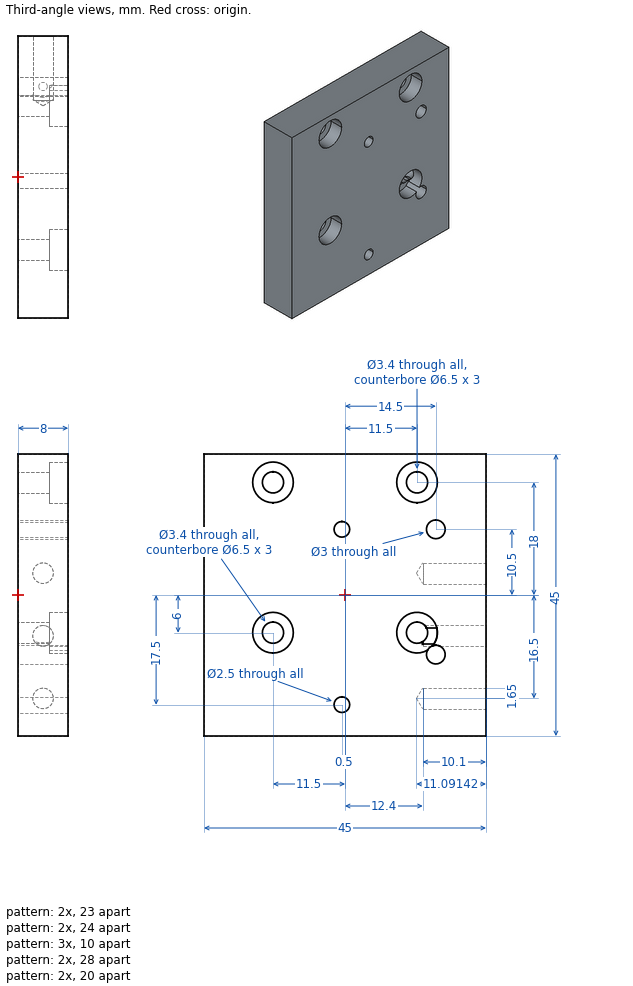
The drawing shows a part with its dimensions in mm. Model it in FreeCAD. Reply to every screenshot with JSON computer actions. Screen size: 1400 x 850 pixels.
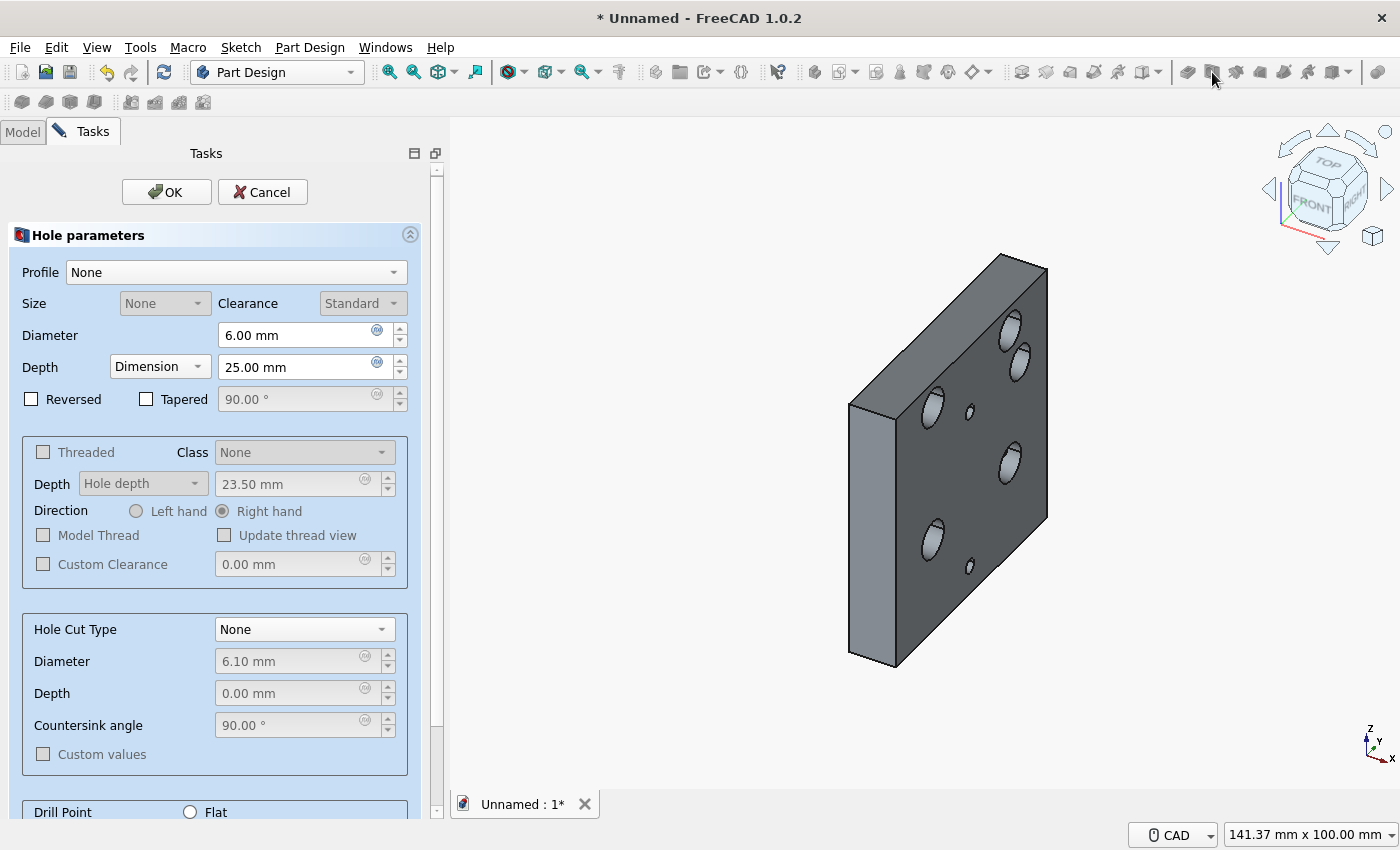
{"action": "triple_click", "coordinate": [305, 335]}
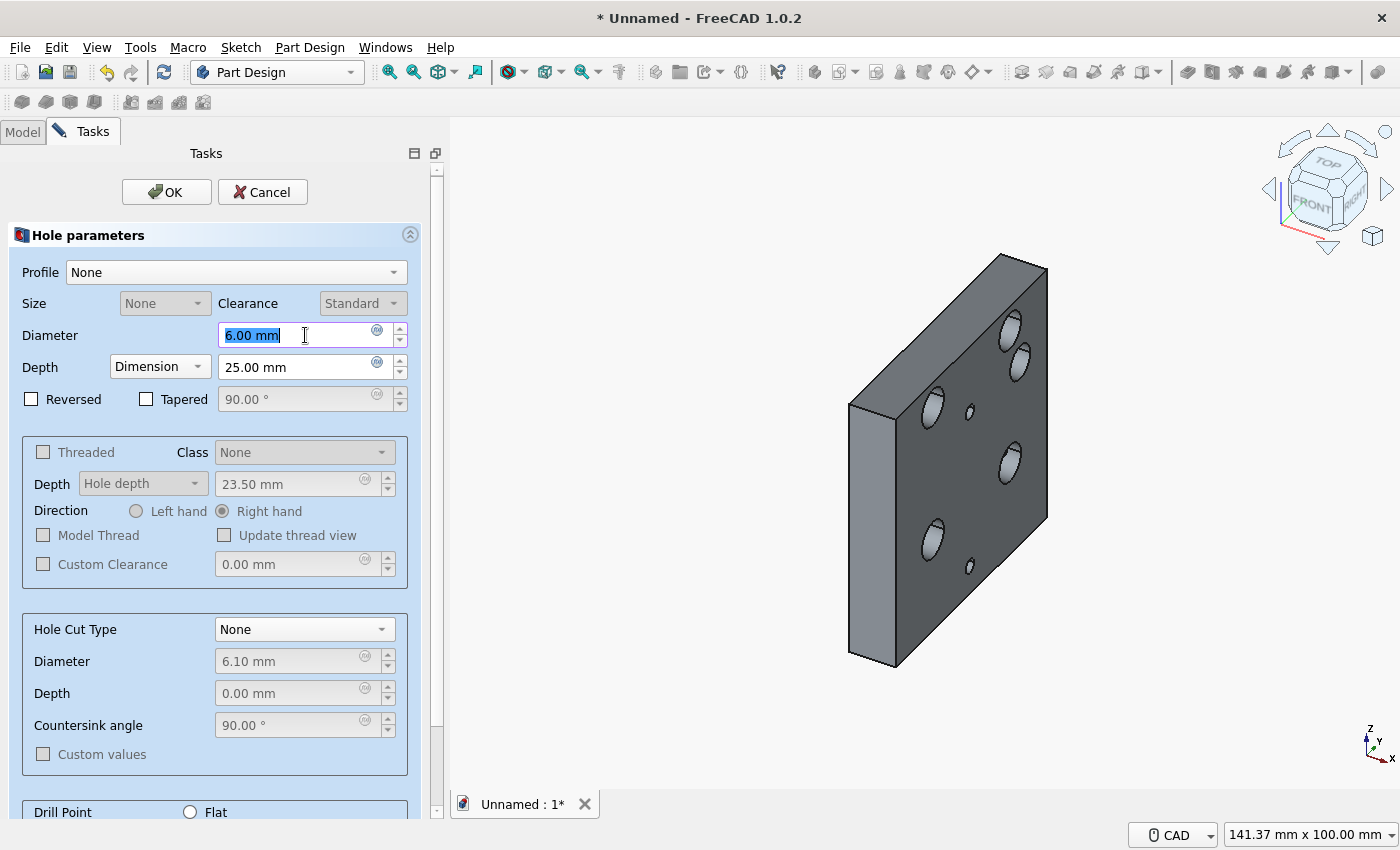
{"action": "type", "text": "3"}
{"action": "key", "text": "Tab"}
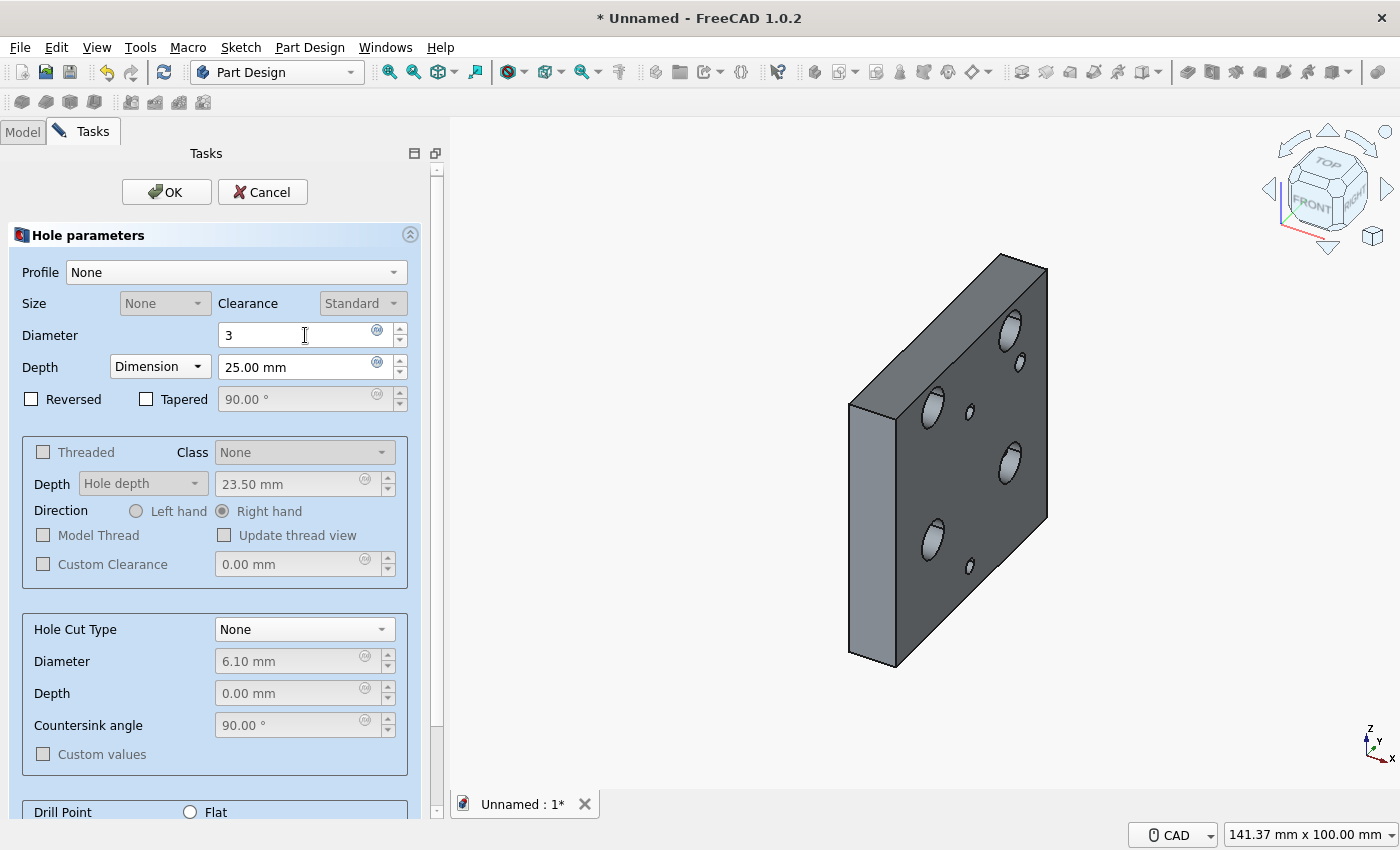
{"action": "left_click", "coordinate": [161, 366]}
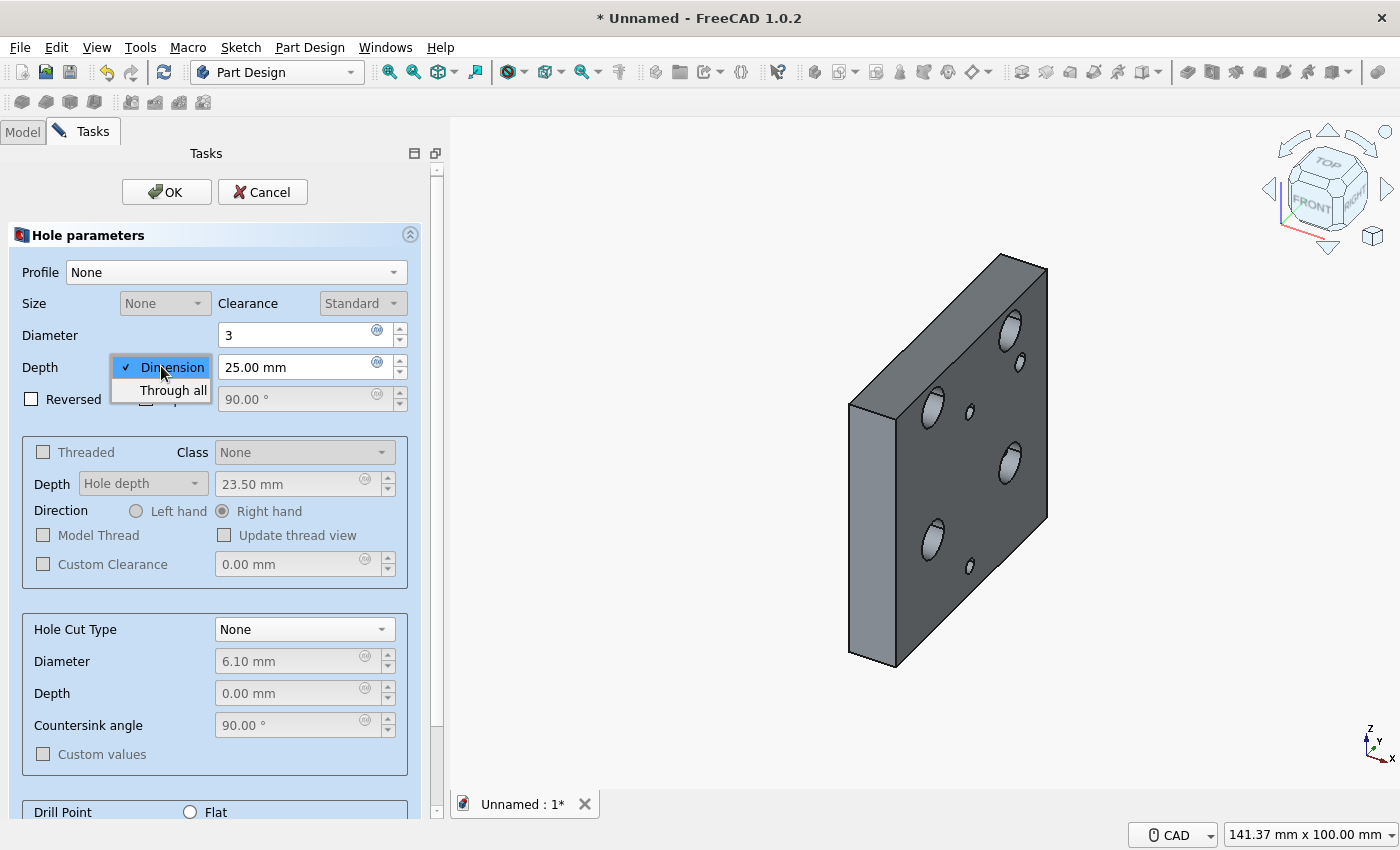
{"action": "left_click", "coordinate": [160, 390]}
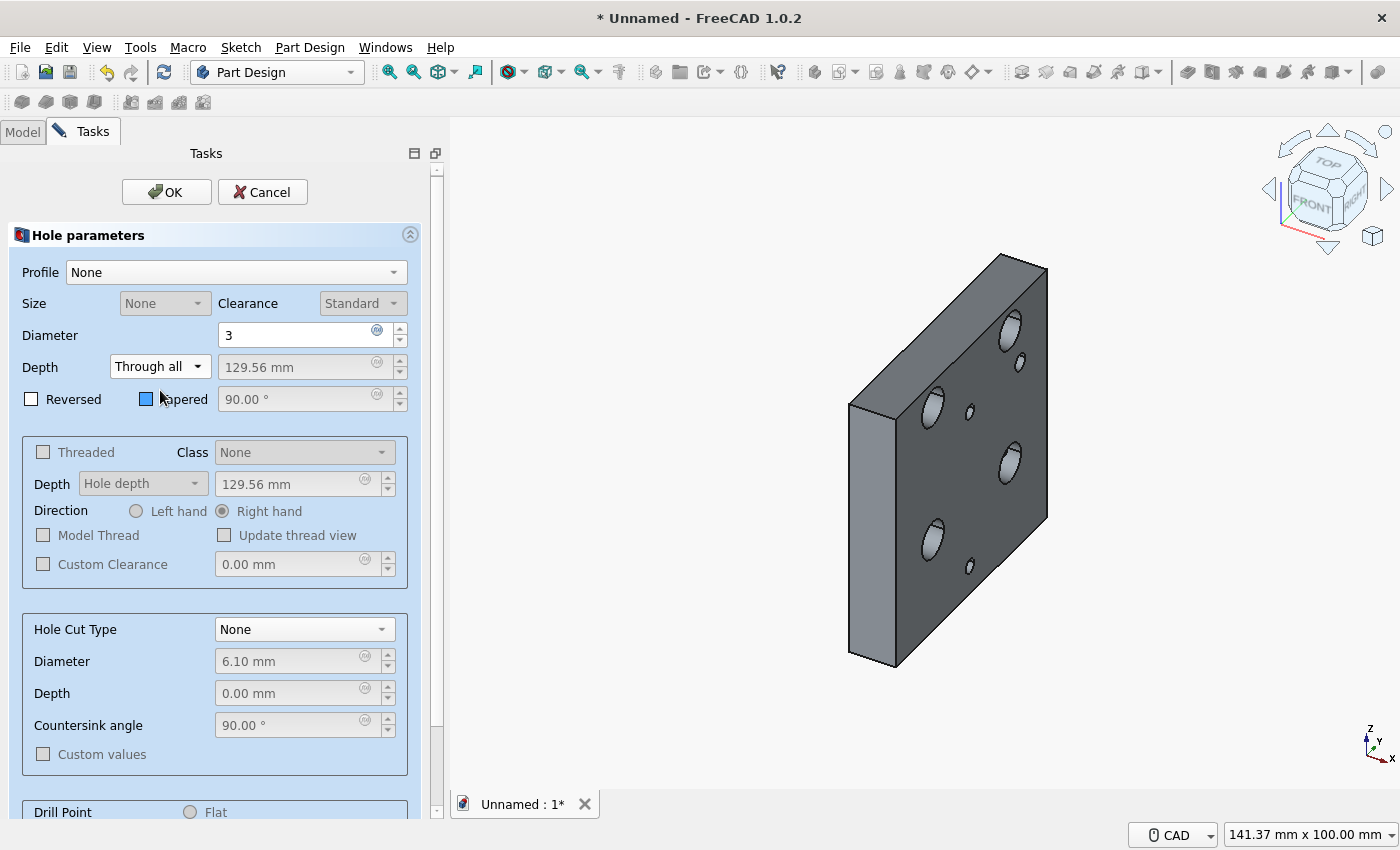
{"action": "left_click", "coordinate": [167, 192]}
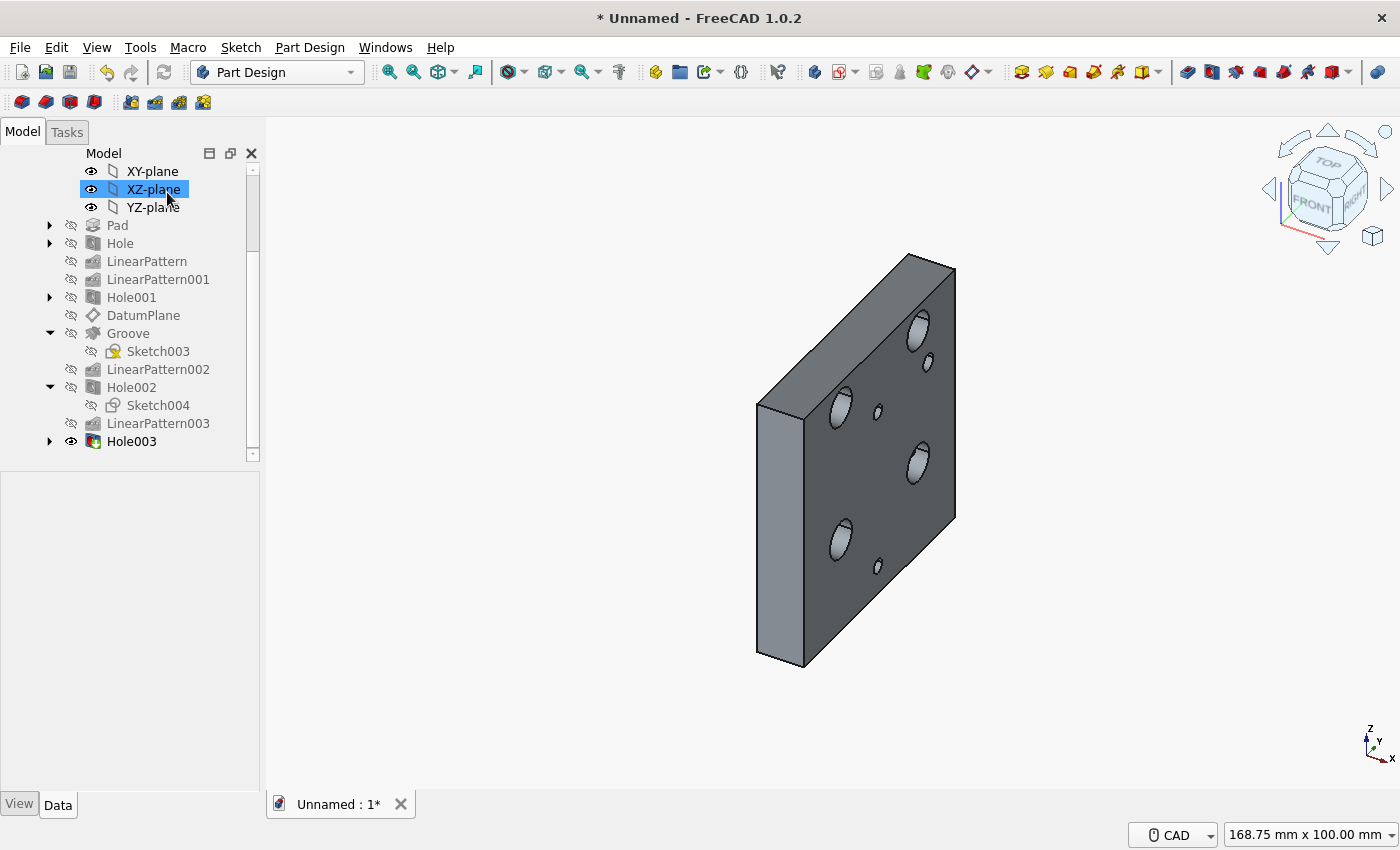
{"action": "left_click", "coordinate": [116, 441]}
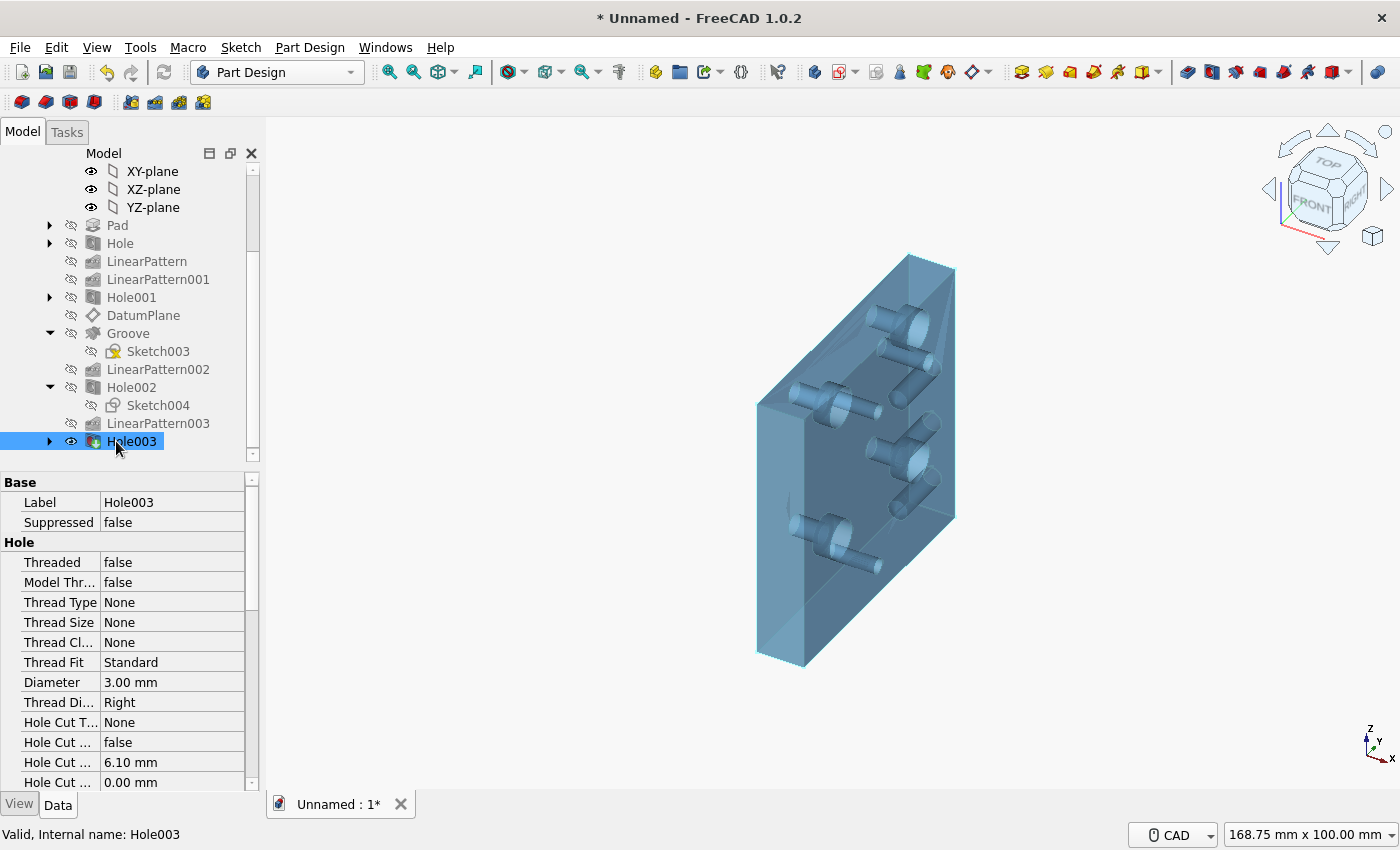
{"action": "left_click", "coordinate": [156, 102]}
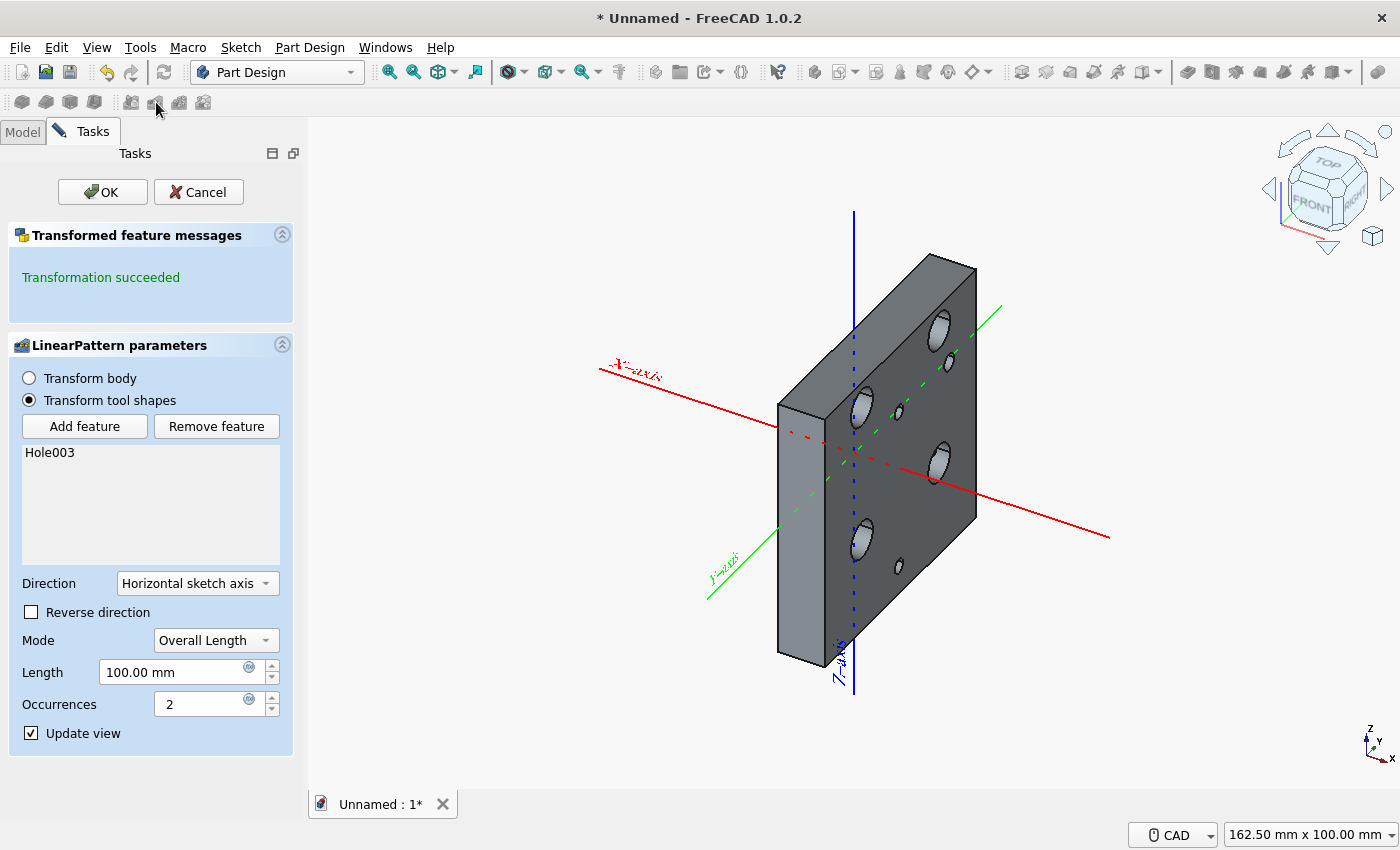
{"action": "left_click", "coordinate": [198, 584]}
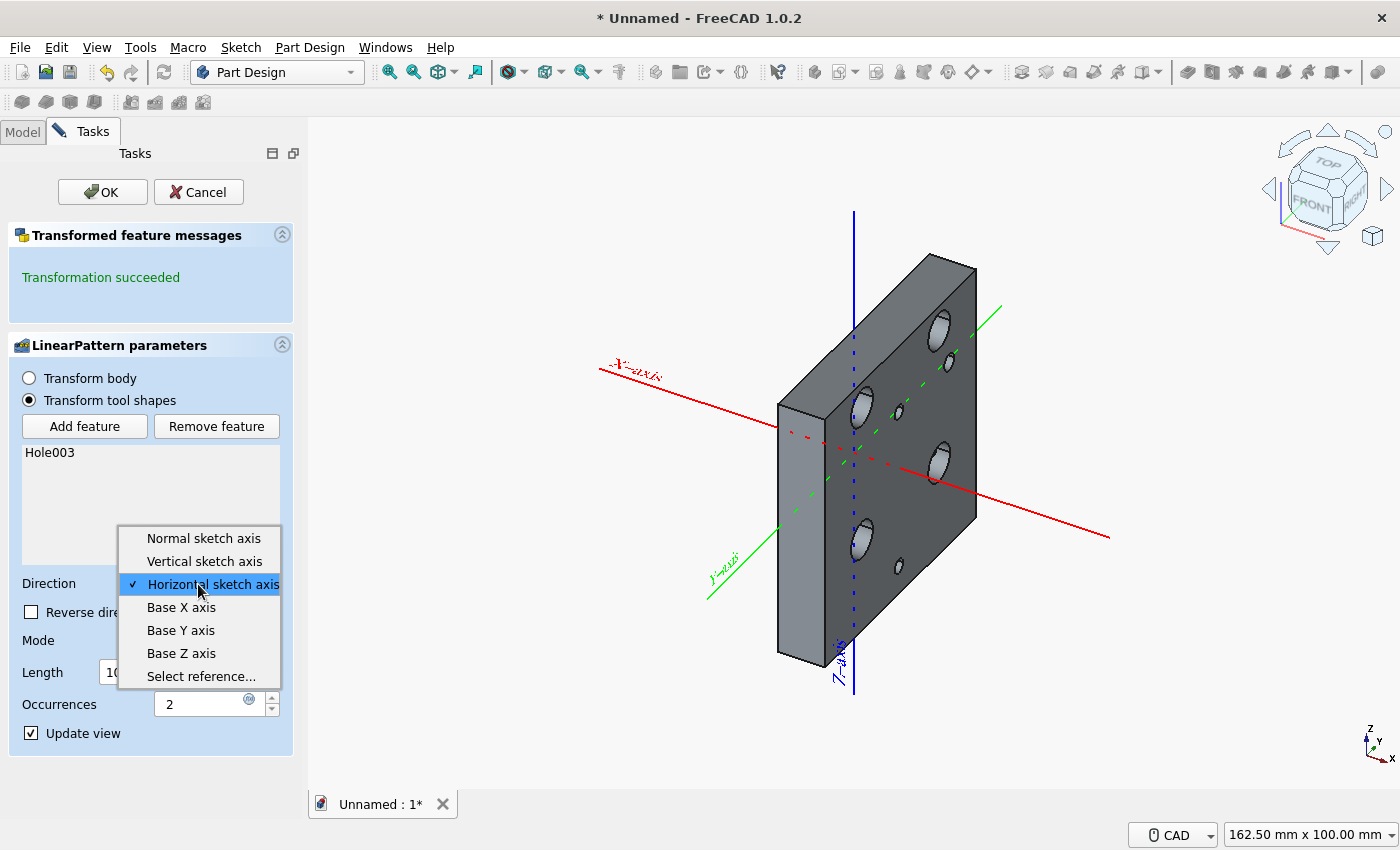
{"action": "left_click", "coordinate": [198, 654]}